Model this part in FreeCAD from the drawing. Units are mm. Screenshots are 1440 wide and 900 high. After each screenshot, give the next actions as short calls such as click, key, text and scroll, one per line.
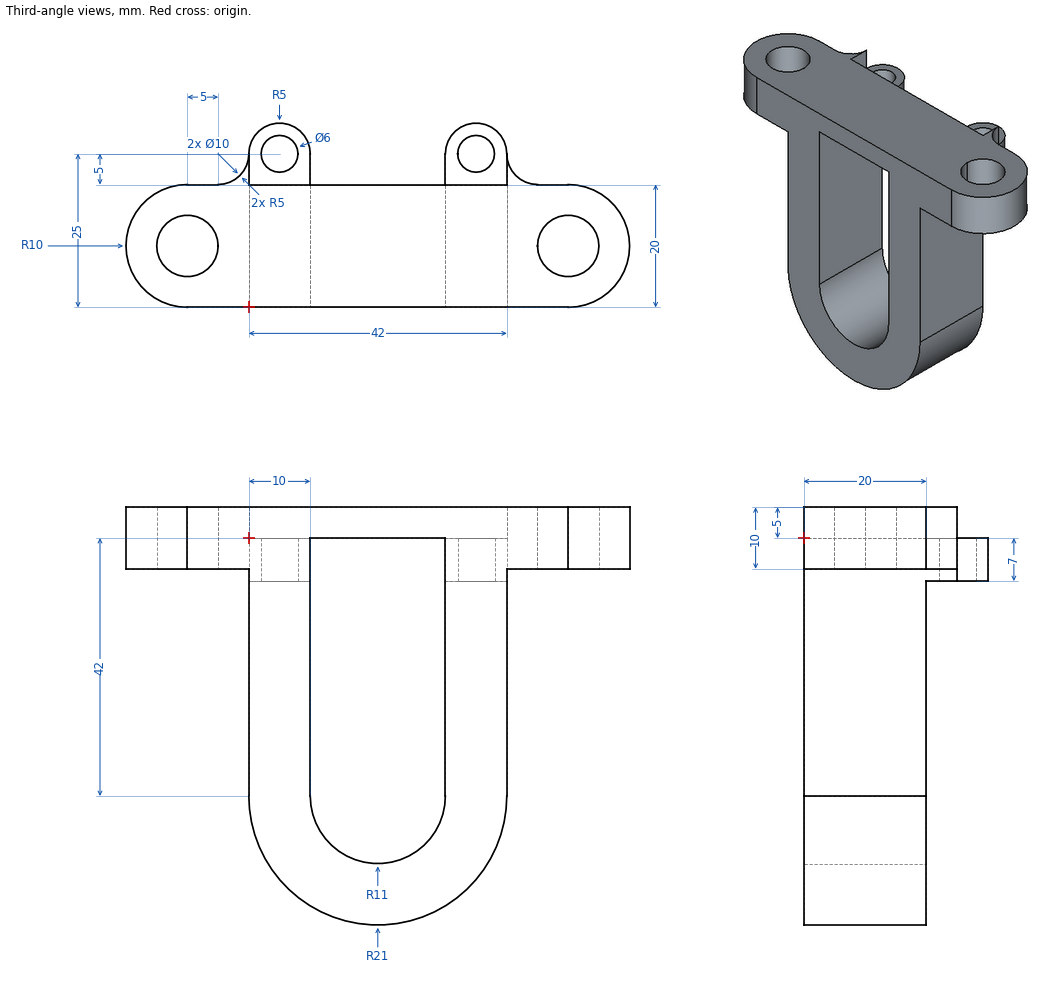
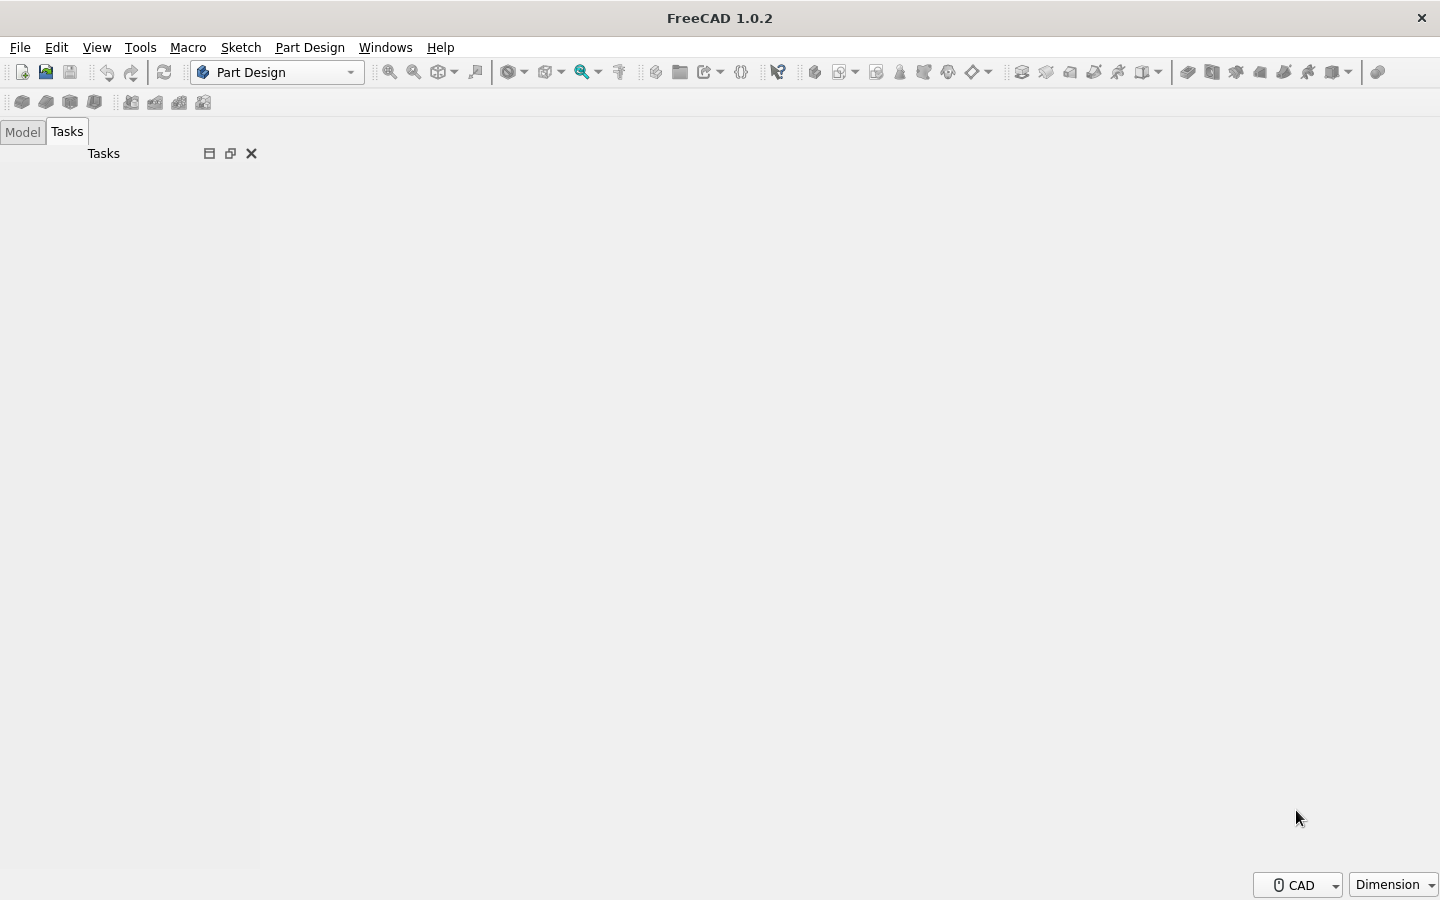
click(22, 72)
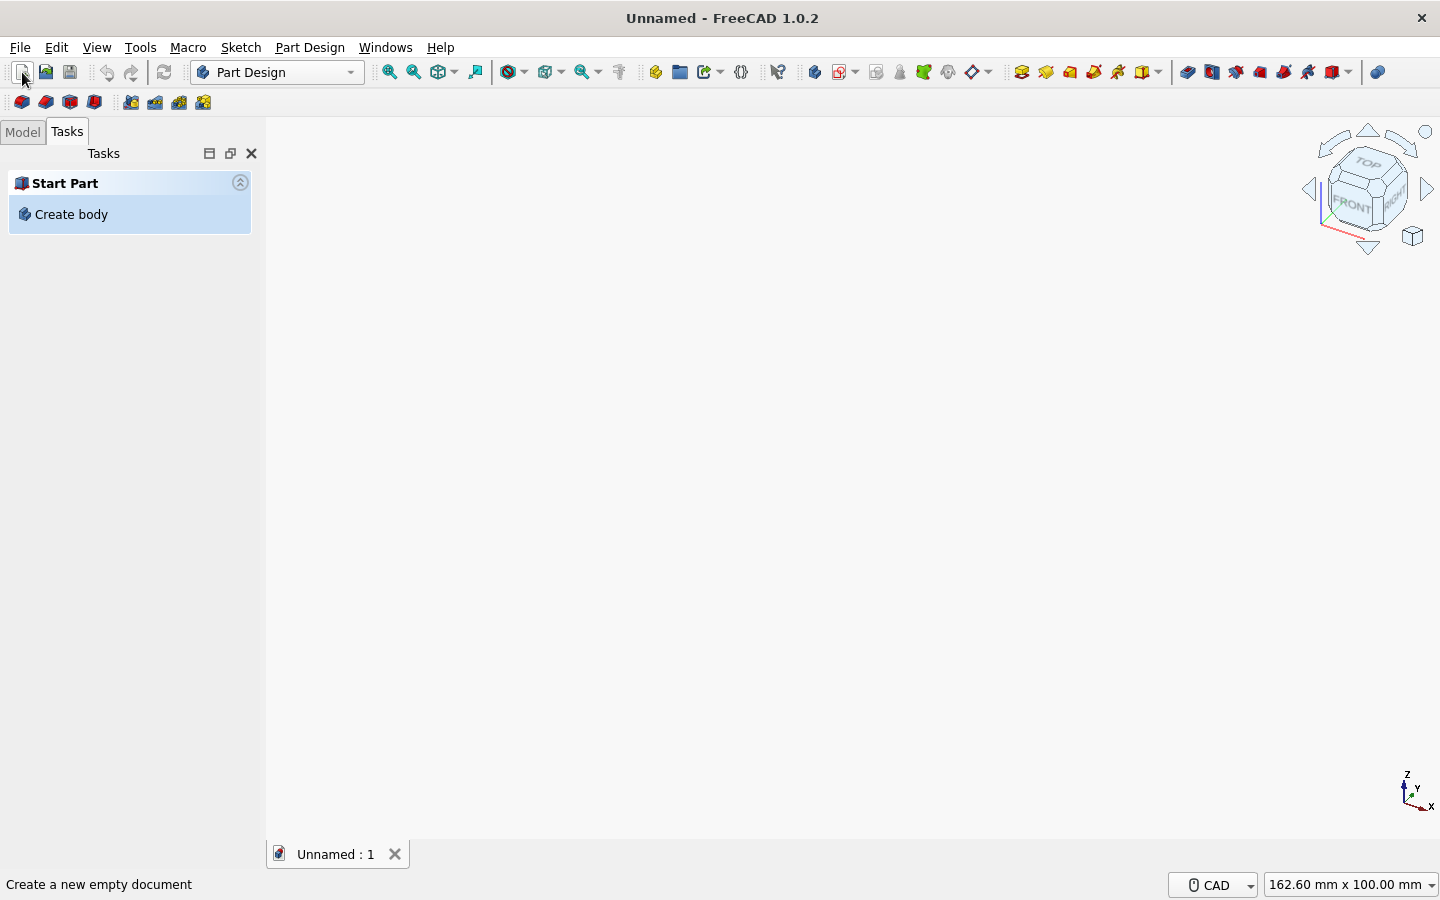
click(840, 72)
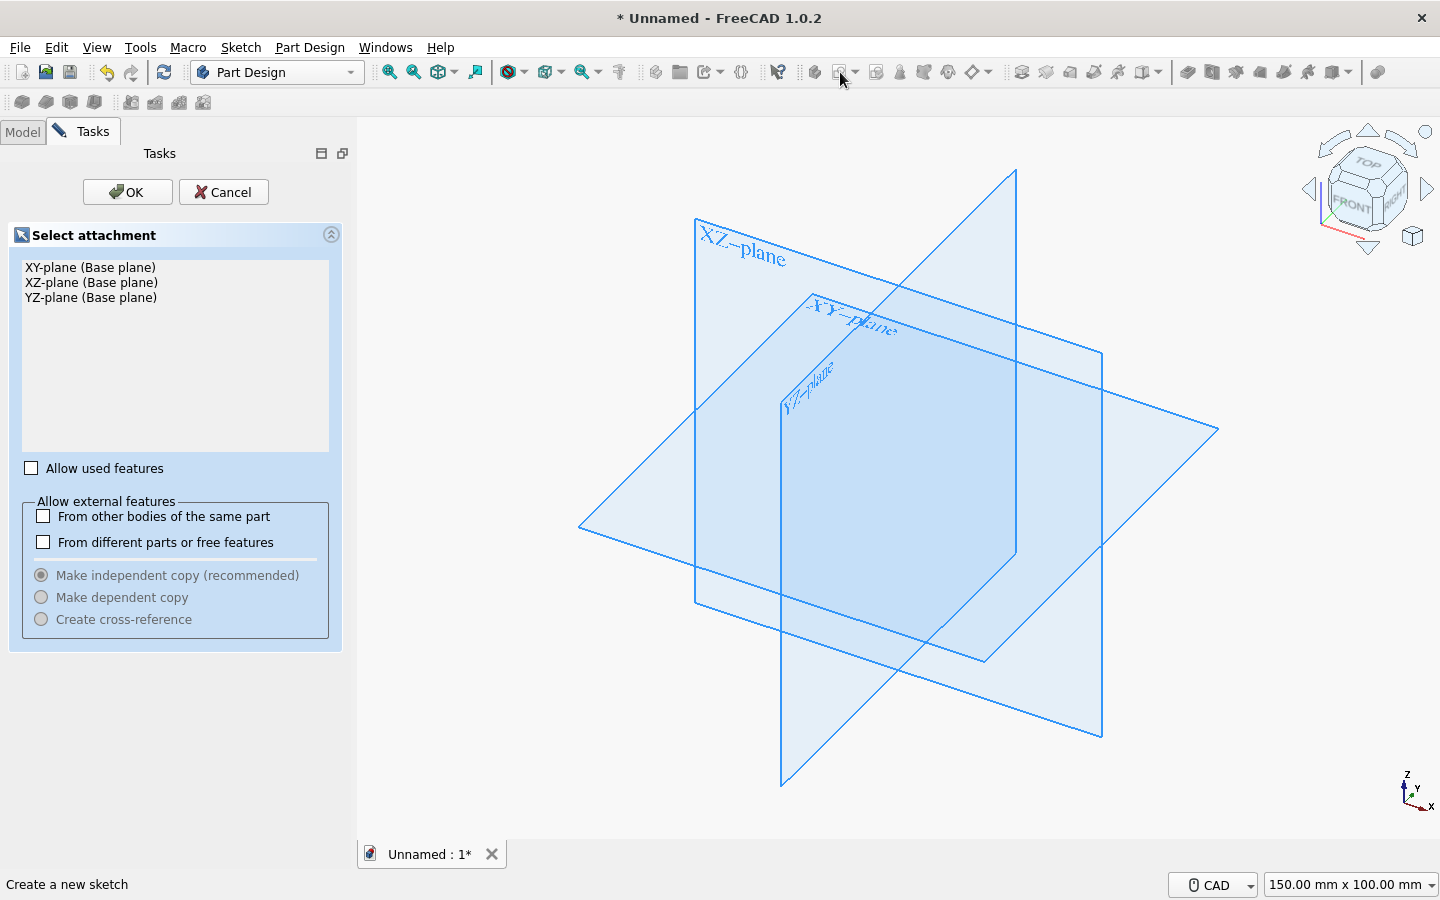
click(82, 268)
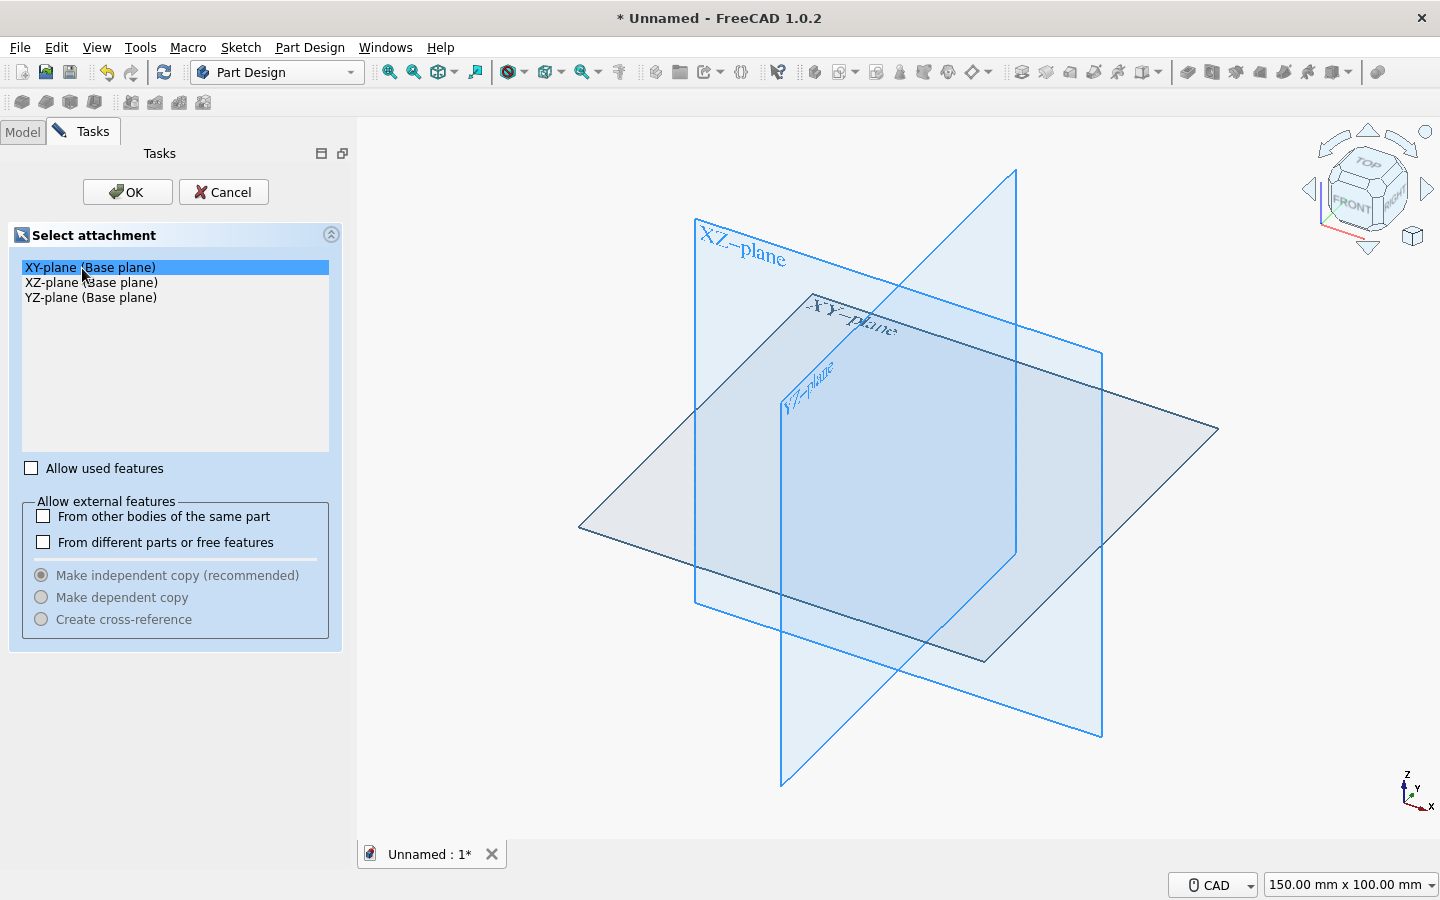
click(128, 192)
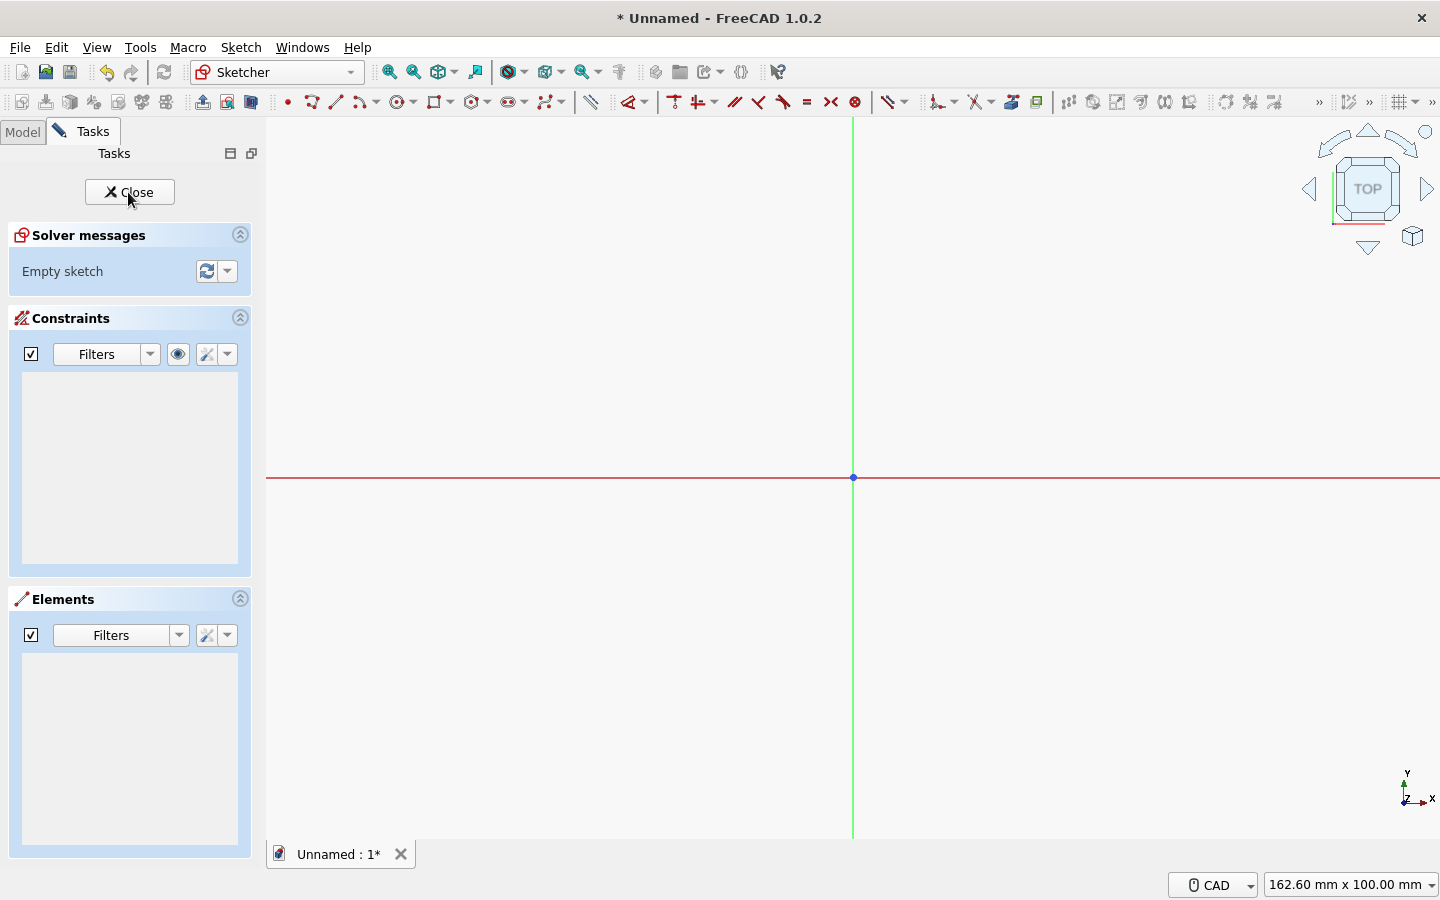
scroll(1184, 347, up, 4)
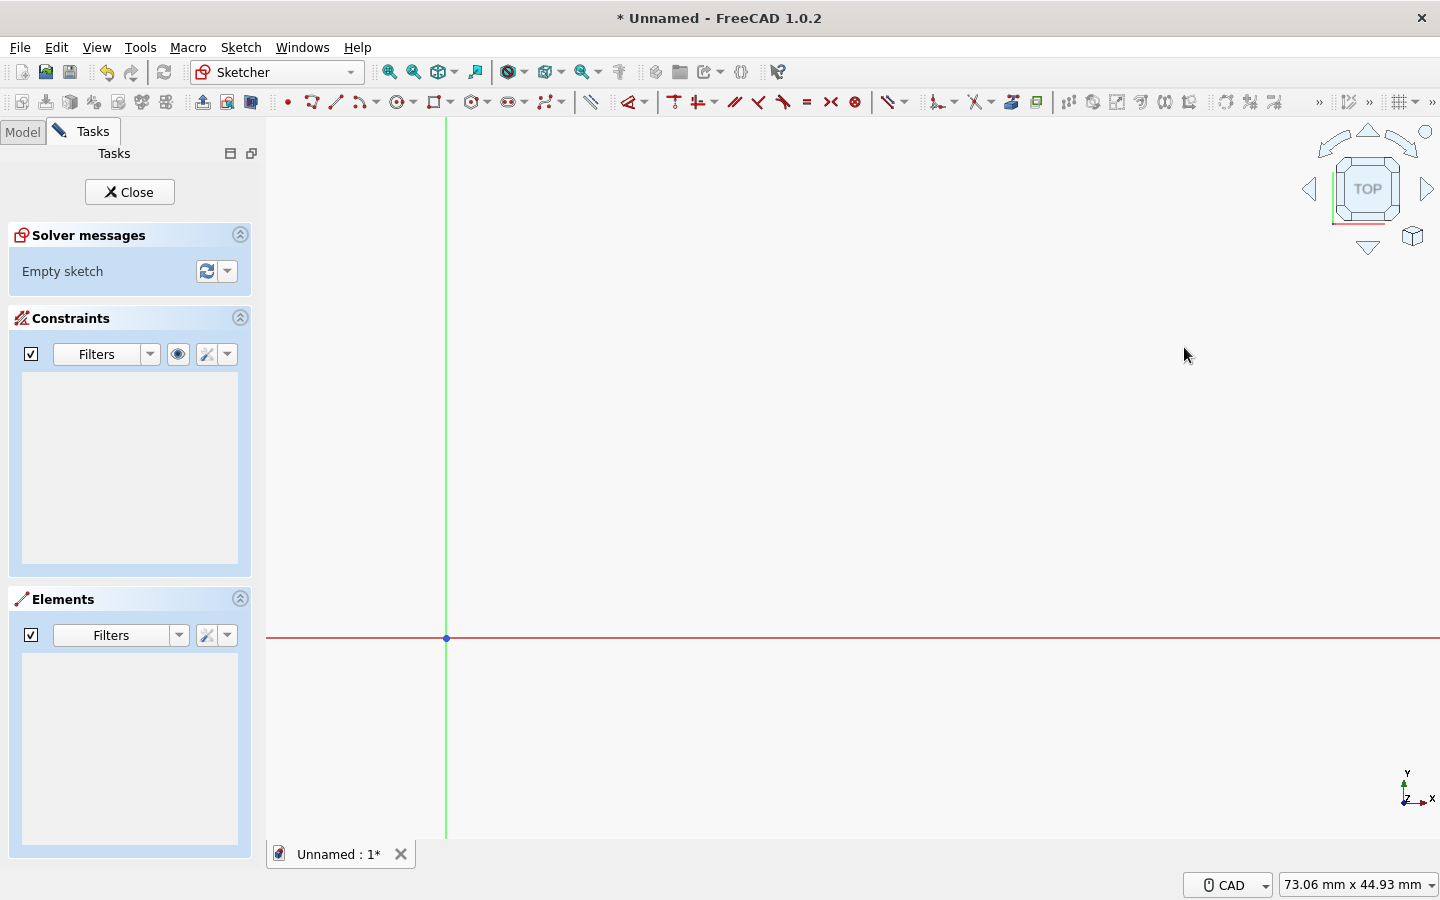
click(434, 102)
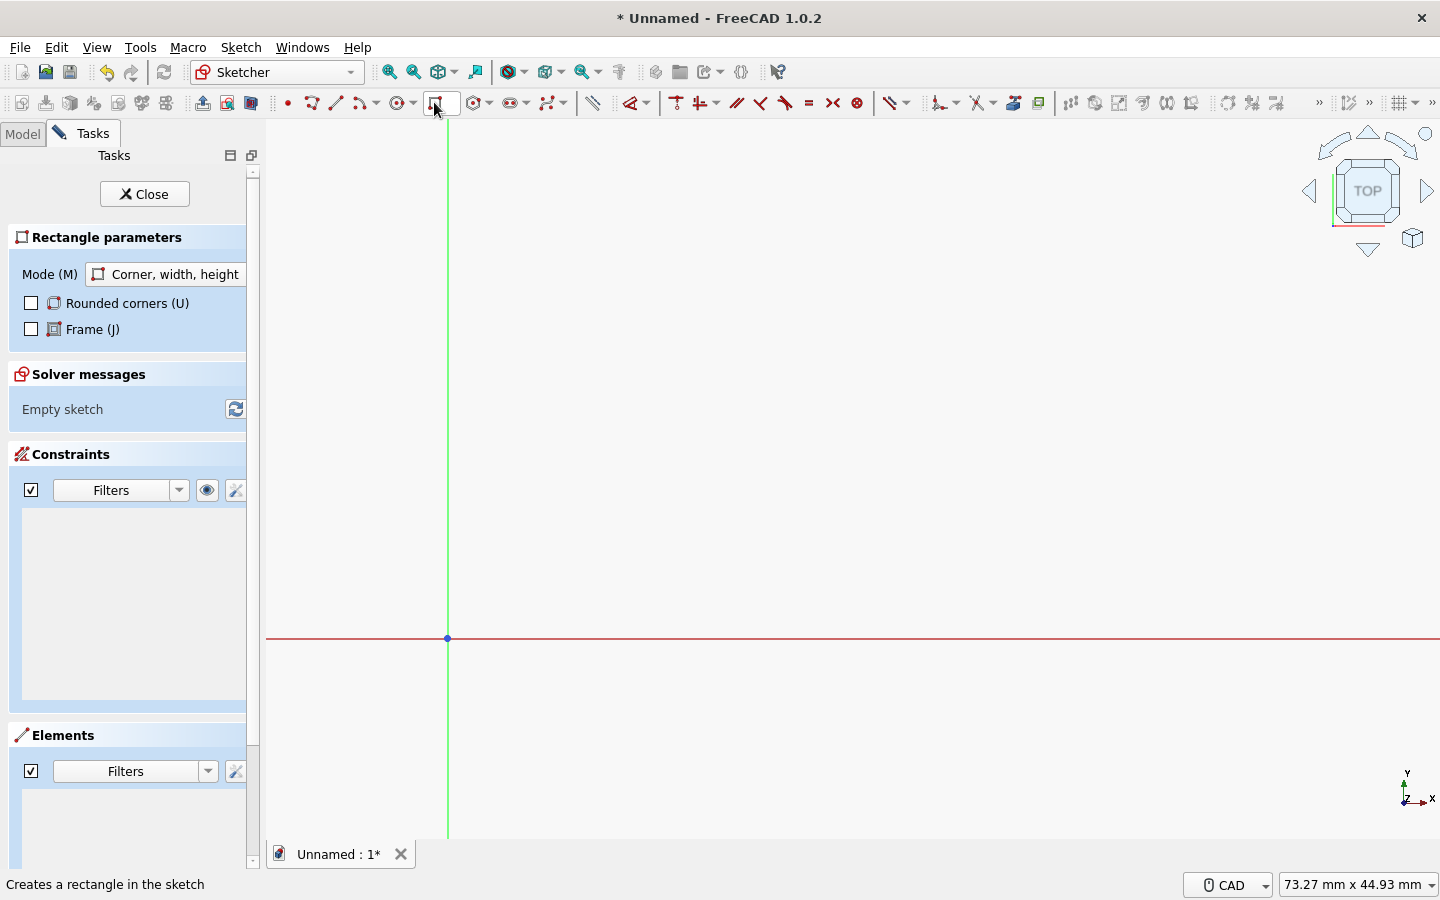
click(448, 639)
click(1121, 318)
key(Escape)